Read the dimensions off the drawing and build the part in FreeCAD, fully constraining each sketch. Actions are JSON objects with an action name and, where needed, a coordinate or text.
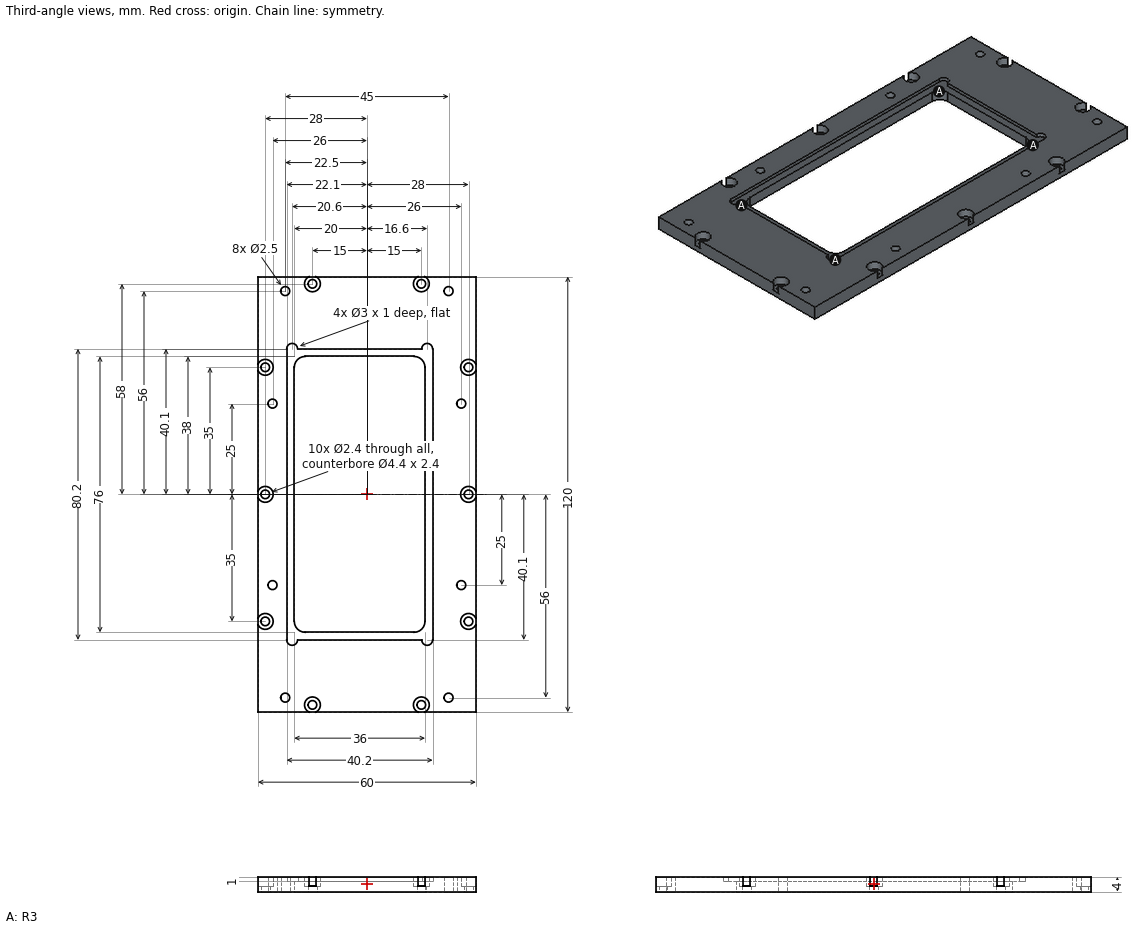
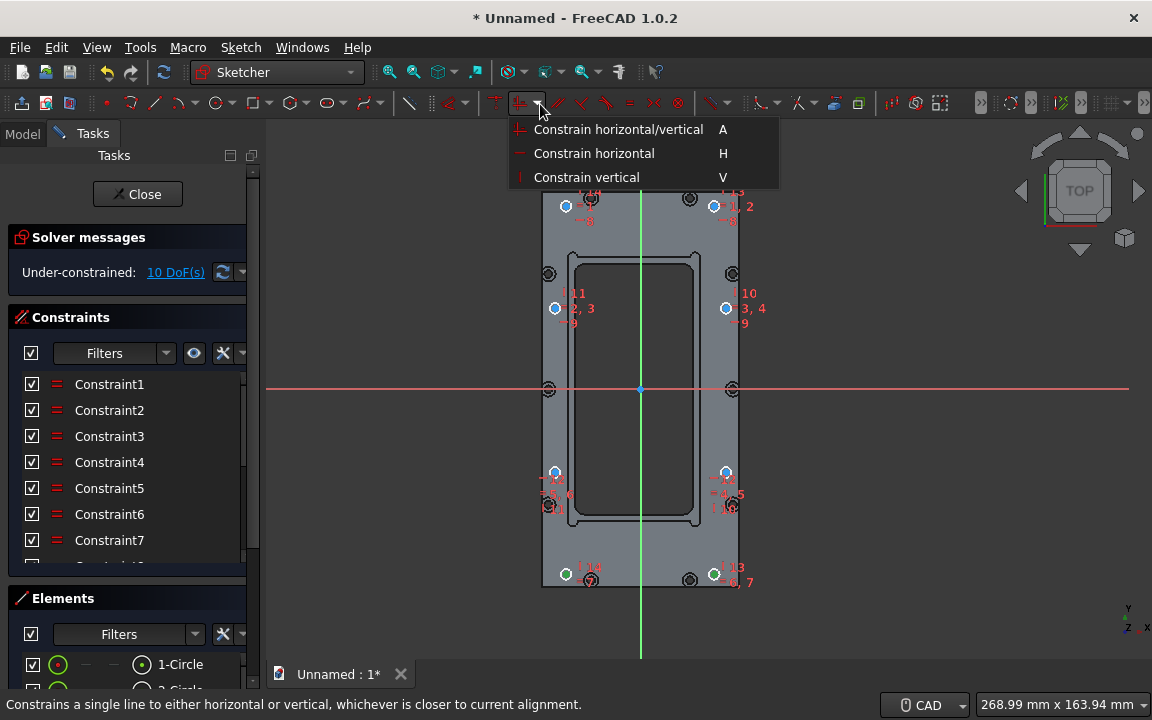
{"action": "left_click", "coordinate": [644, 153]}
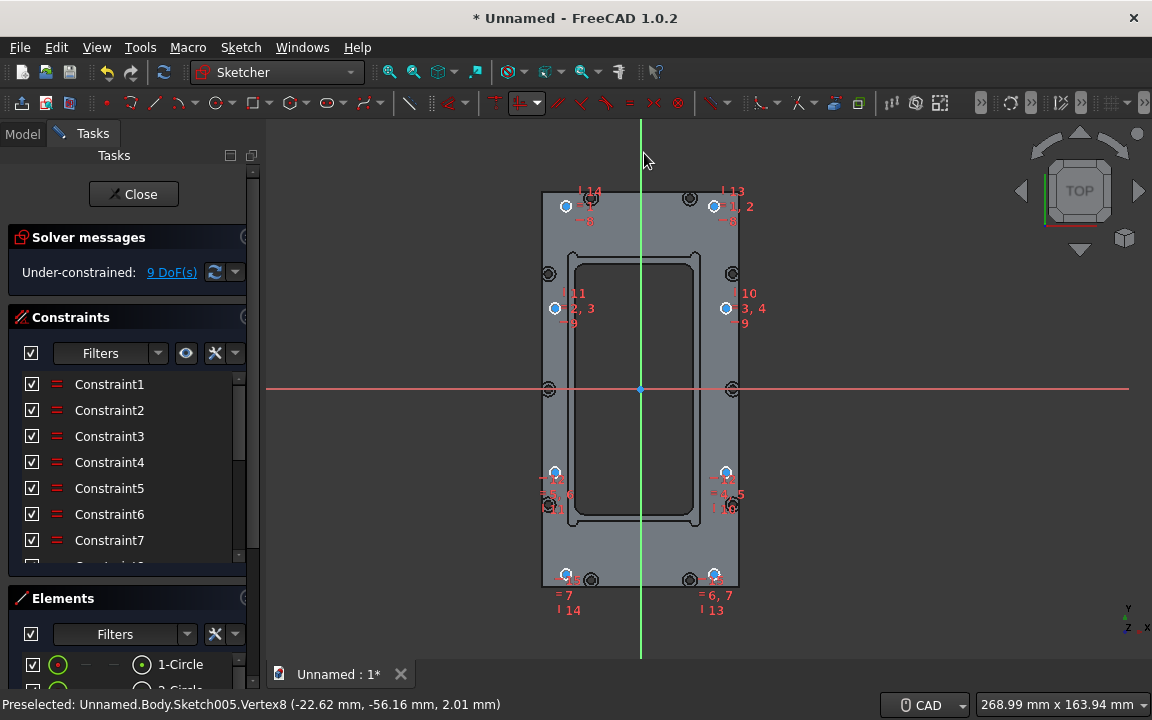
{"action": "left_click", "coordinate": [448, 104]}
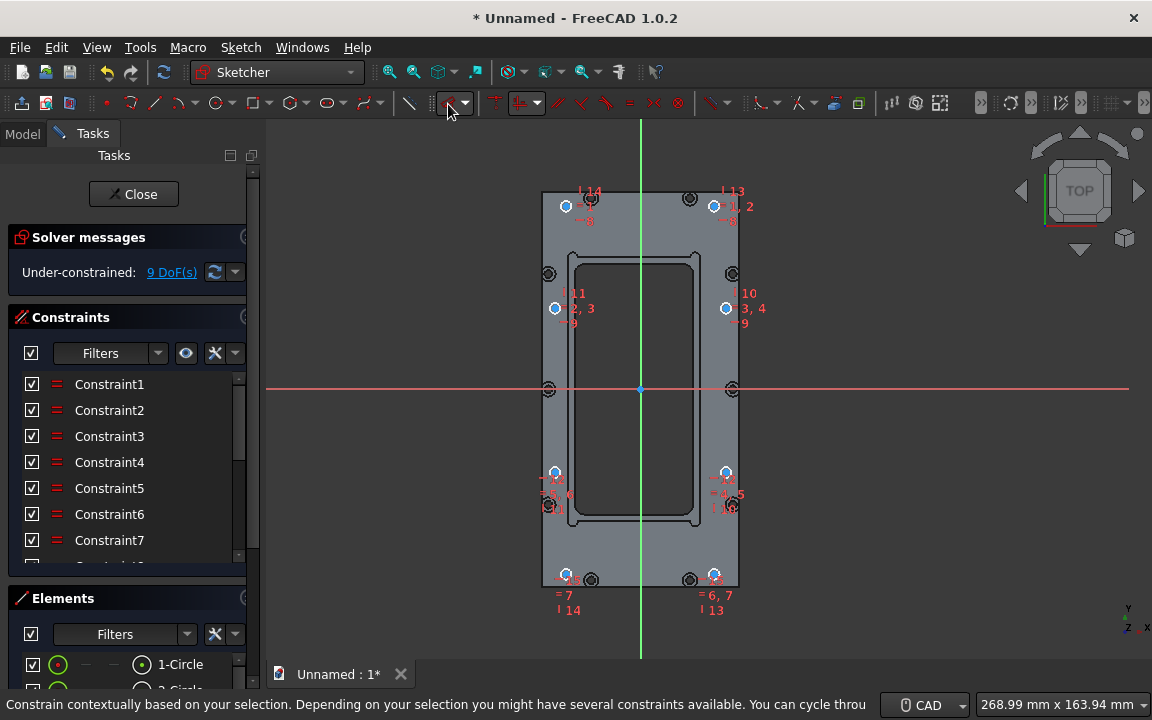
{"action": "scroll", "coordinate": [561, 206], "scroll_direction": "up", "scroll_amount": 8}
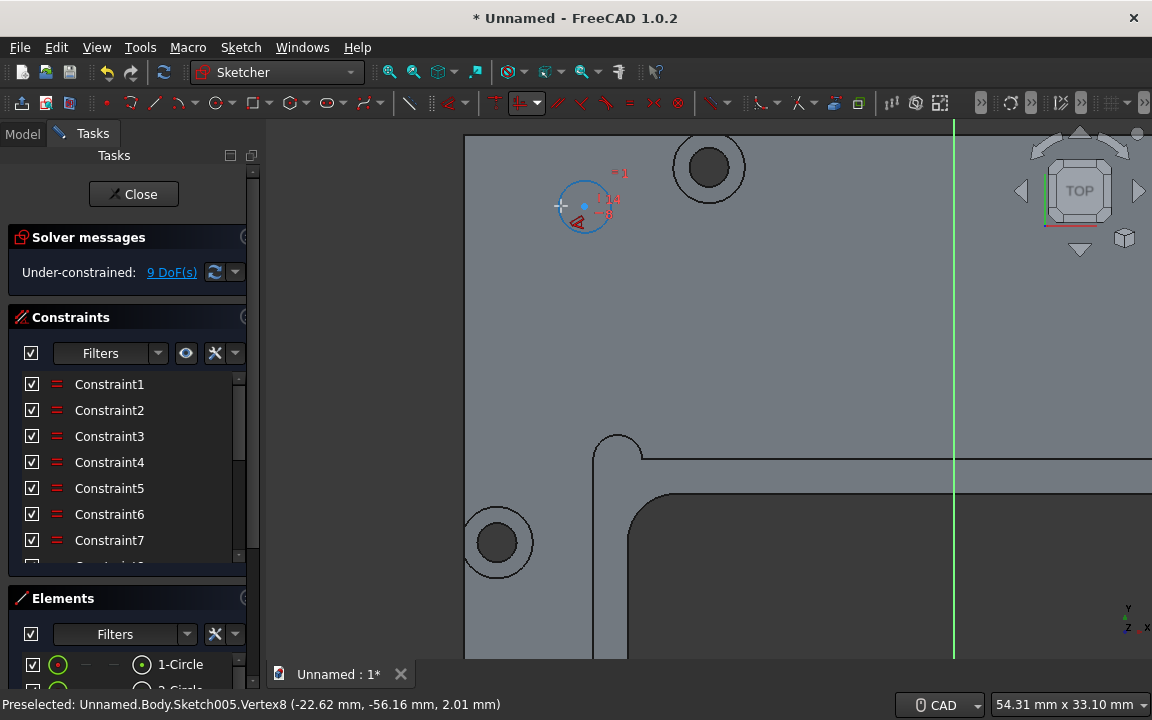
{"action": "left_click", "coordinate": [559, 206]}
{"action": "left_click", "coordinate": [527, 205]}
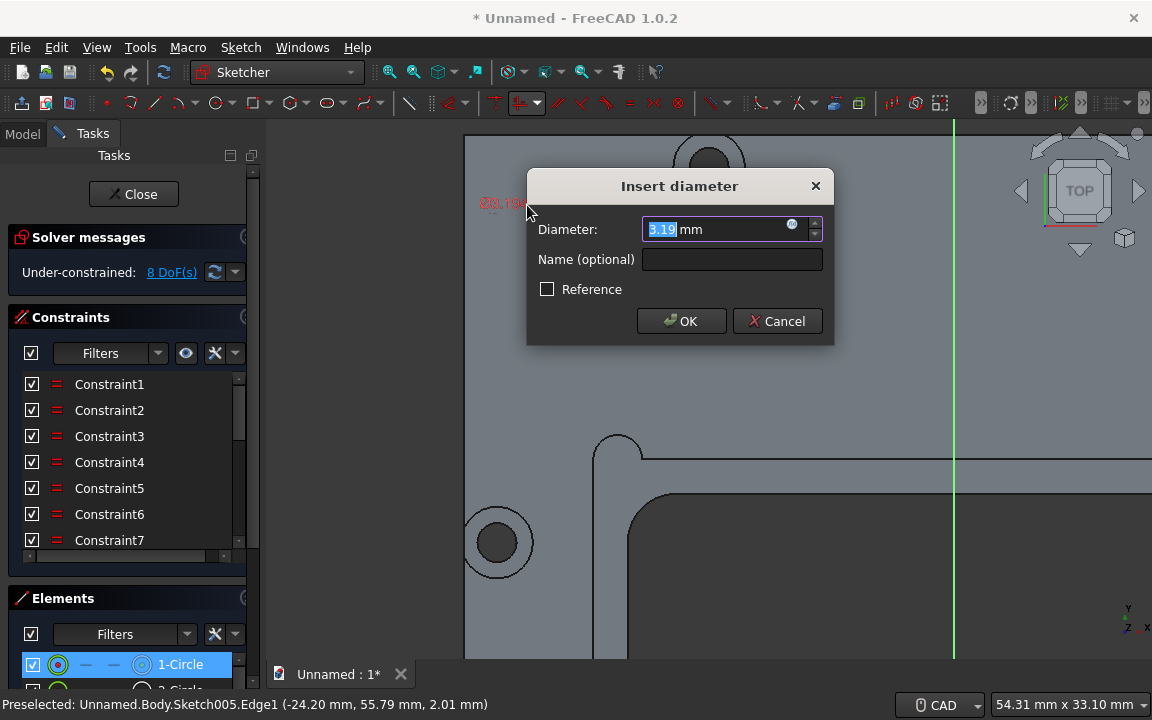
{"action": "type", "text": "2.5"}
{"action": "key", "text": "Return"}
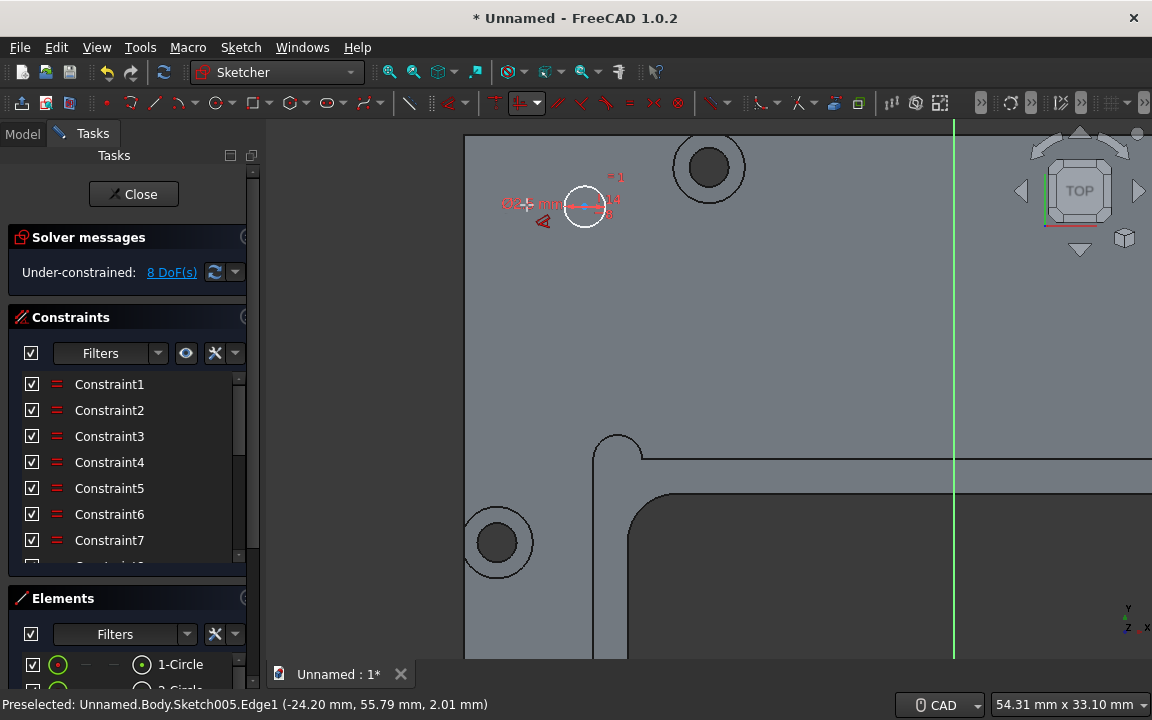
{"action": "scroll", "coordinate": [561, 206], "scroll_direction": "down", "scroll_amount": 8}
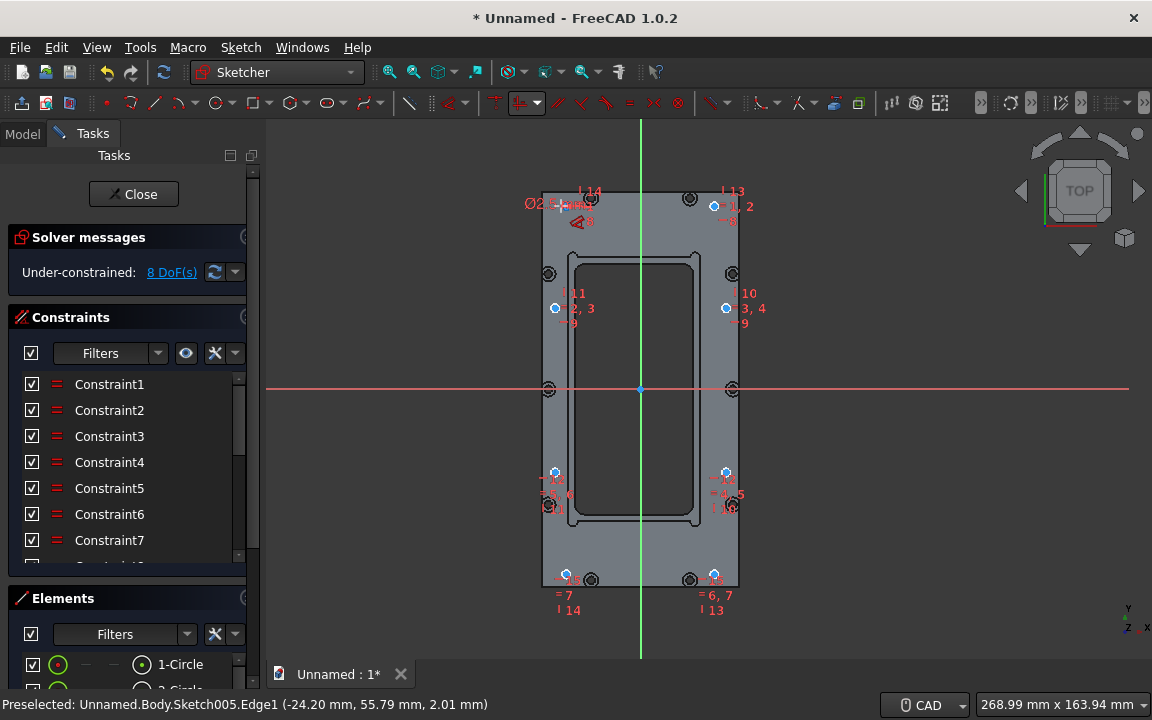
{"action": "left_click", "coordinate": [566, 206]}
{"action": "left_click", "coordinate": [532, 298]}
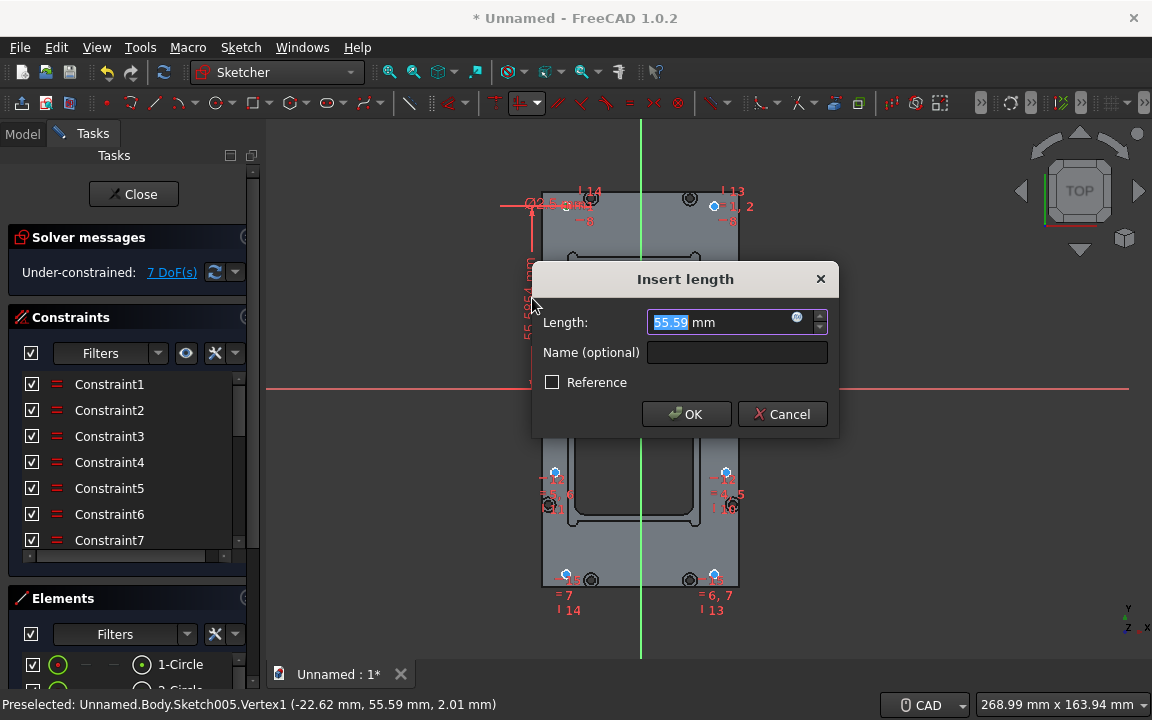
{"action": "type", "text": "56"}
{"action": "key", "text": "Return"}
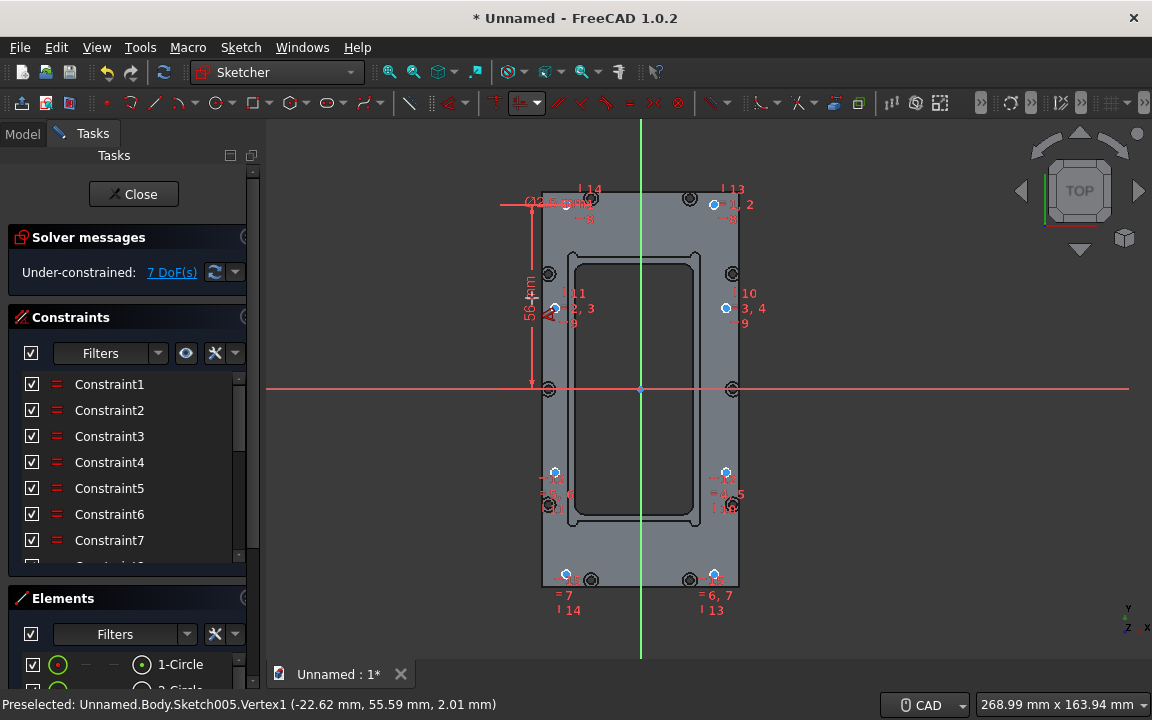
{"action": "left_click", "coordinate": [555, 308]}
{"action": "left_click", "coordinate": [598, 274]}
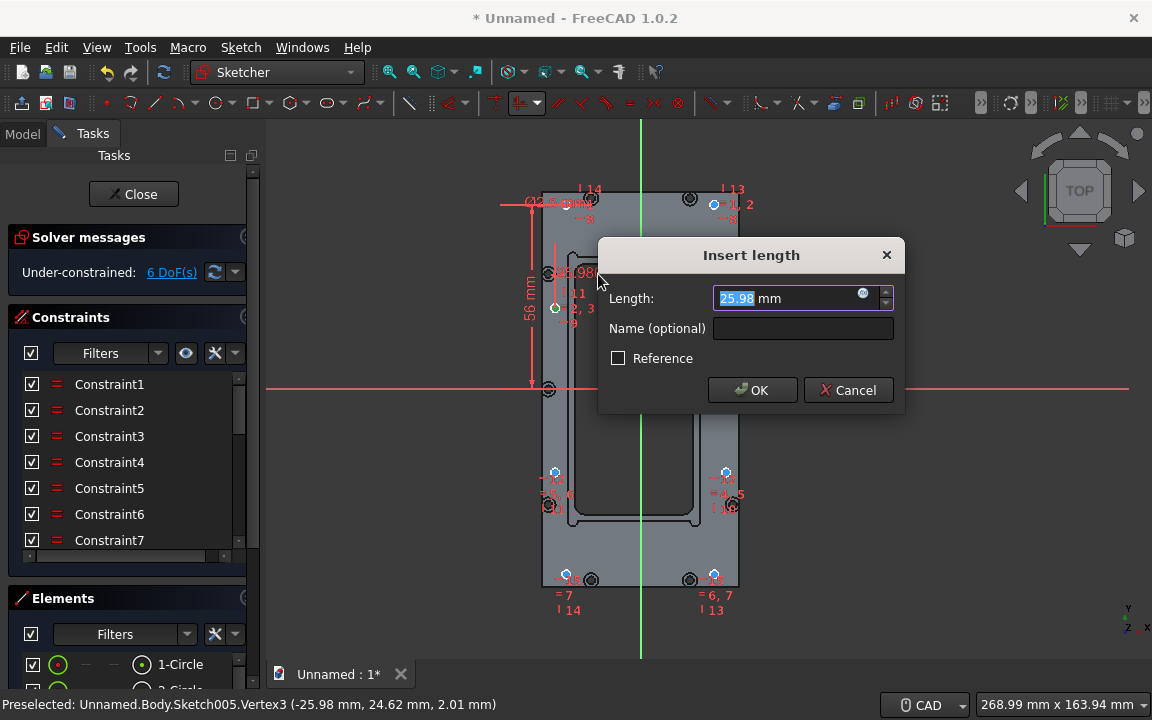
{"action": "type", "text": "26"}
{"action": "key", "text": "Return"}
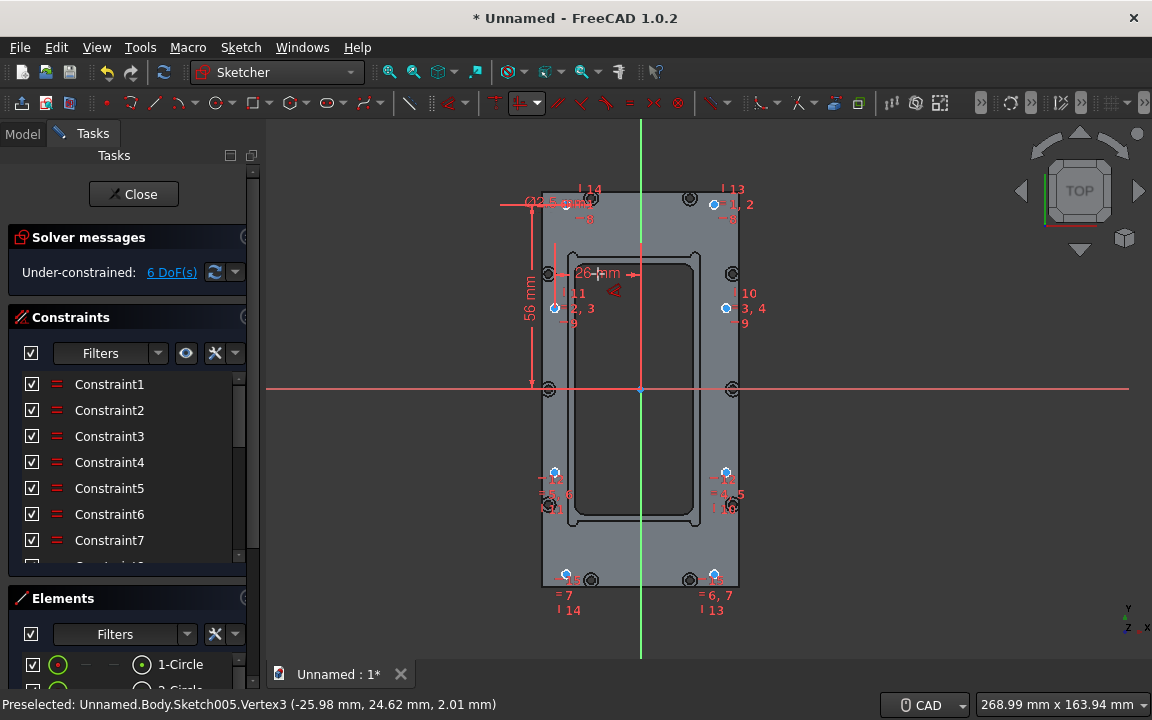
{"action": "left_click", "coordinate": [555, 308]}
{"action": "left_click", "coordinate": [521, 349]}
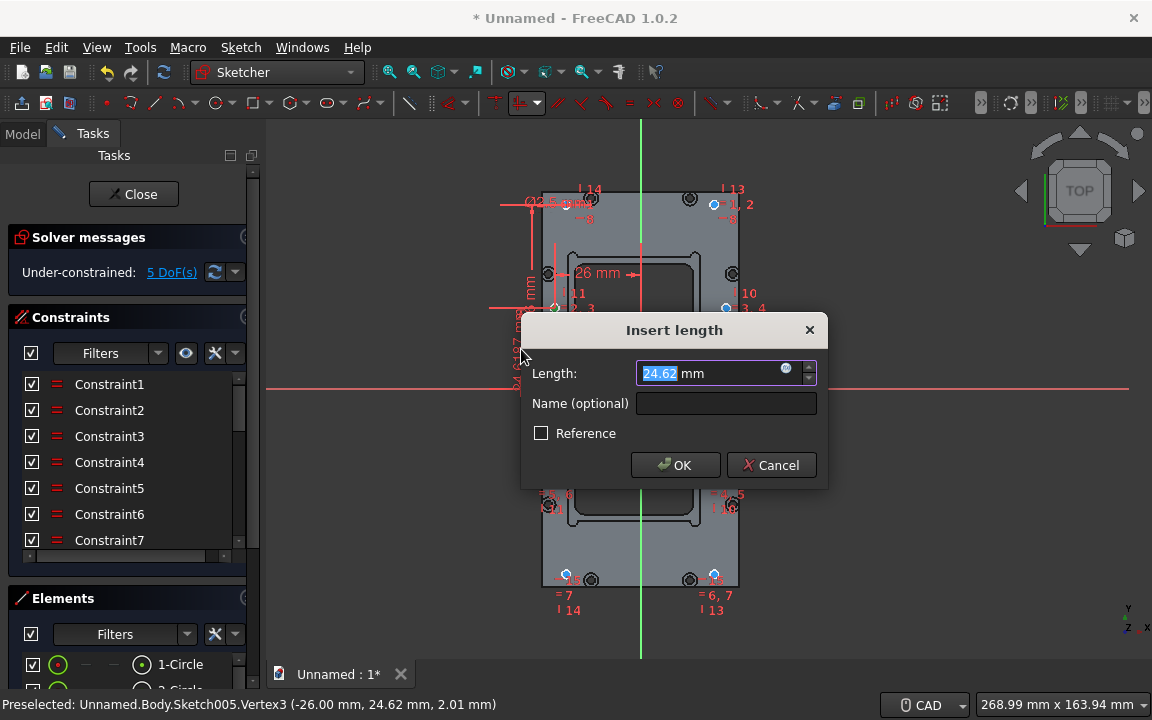
{"action": "type", "text": "25"}
{"action": "key", "text": "Return"}